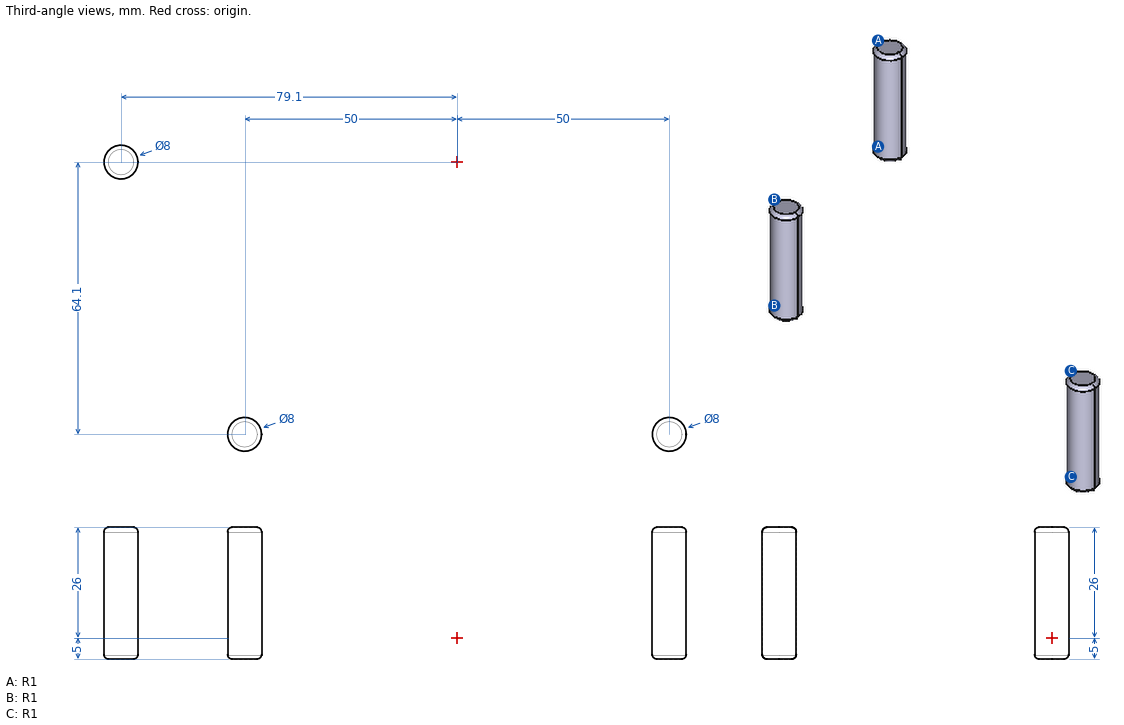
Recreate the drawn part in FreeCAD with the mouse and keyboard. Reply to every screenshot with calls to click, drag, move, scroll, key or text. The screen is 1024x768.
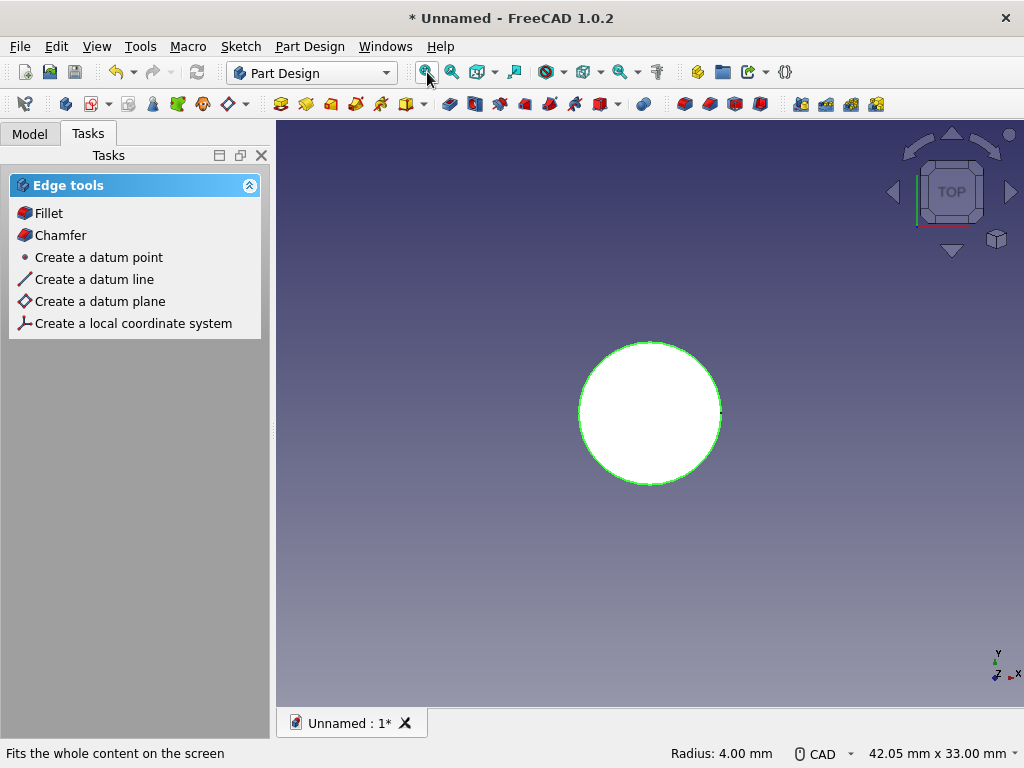
key(1)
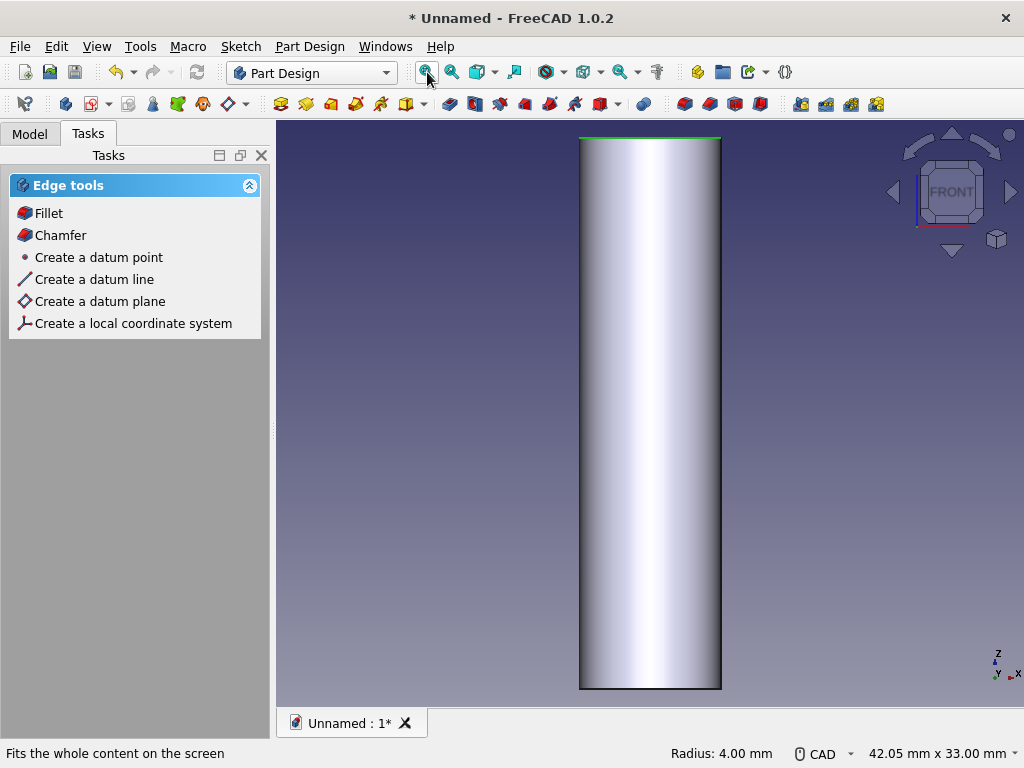
key(3)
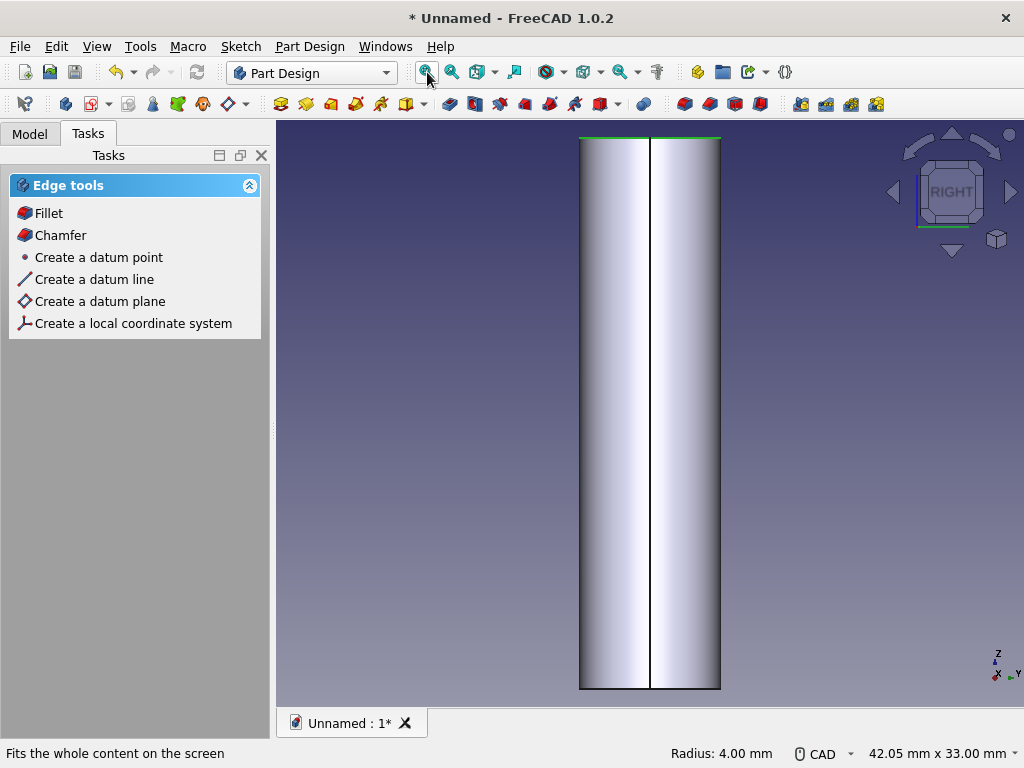
key(5)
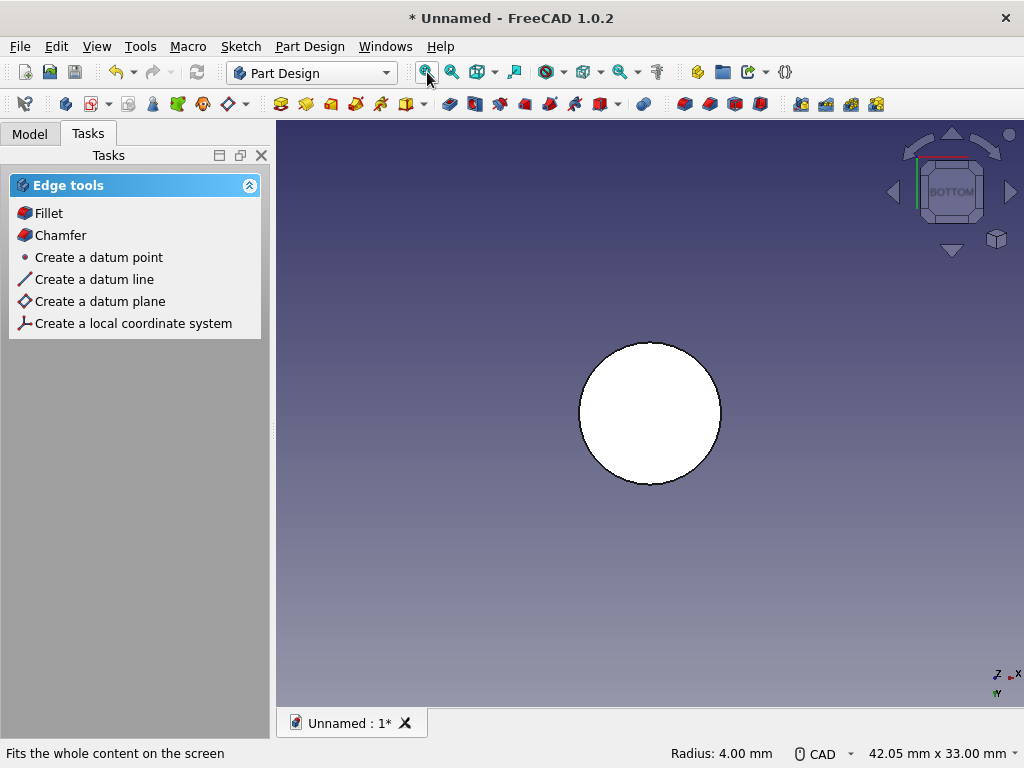
click(427, 72)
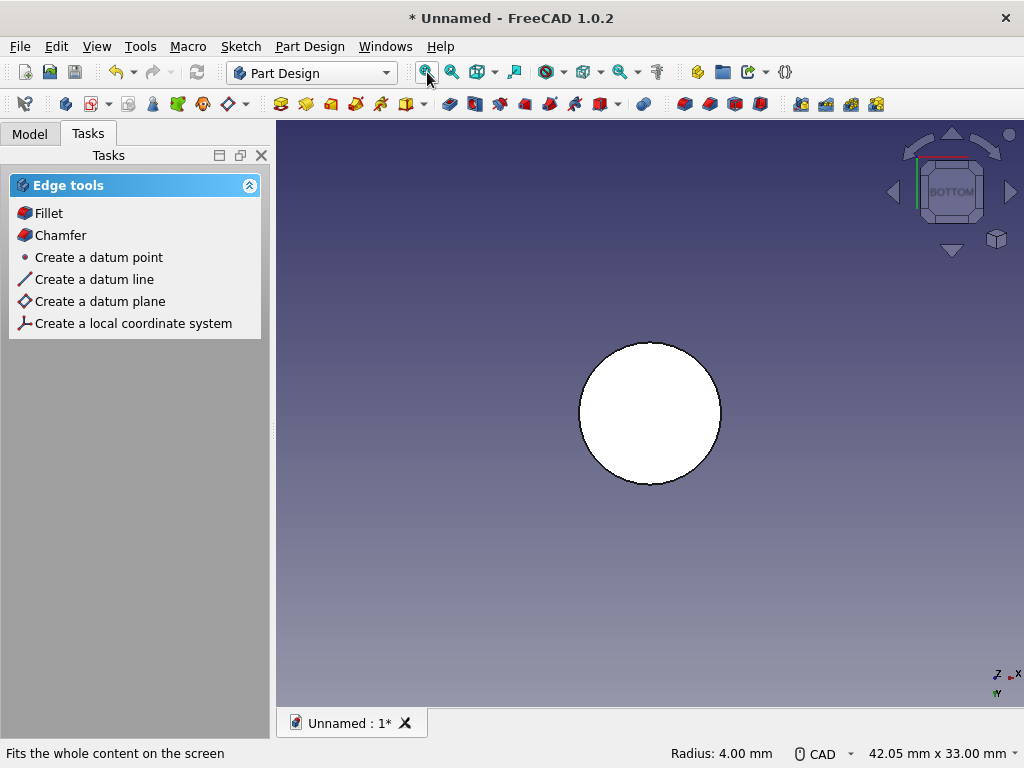
click(579, 412, ctrl)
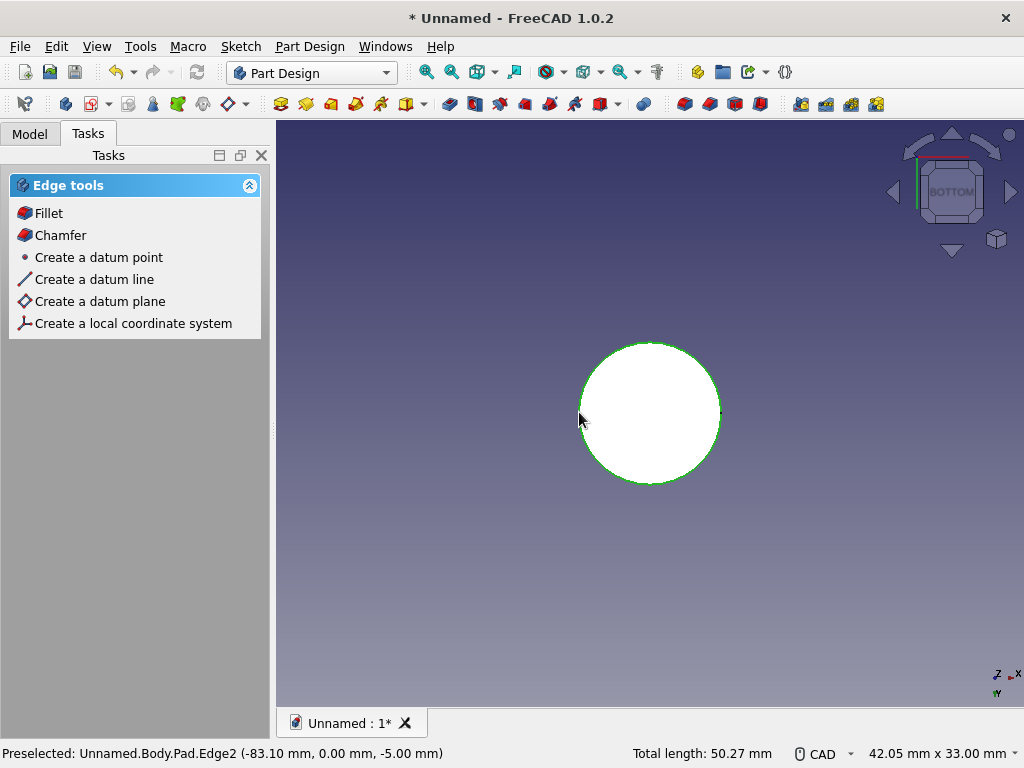
click(685, 104)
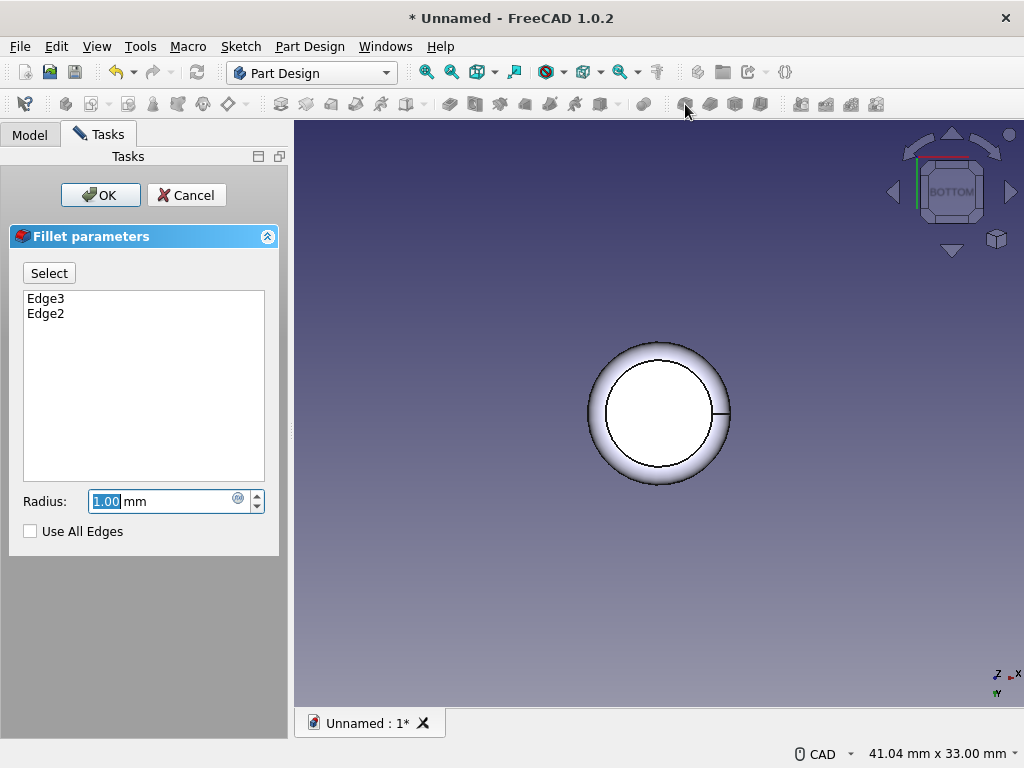
text(1)
key(Tab)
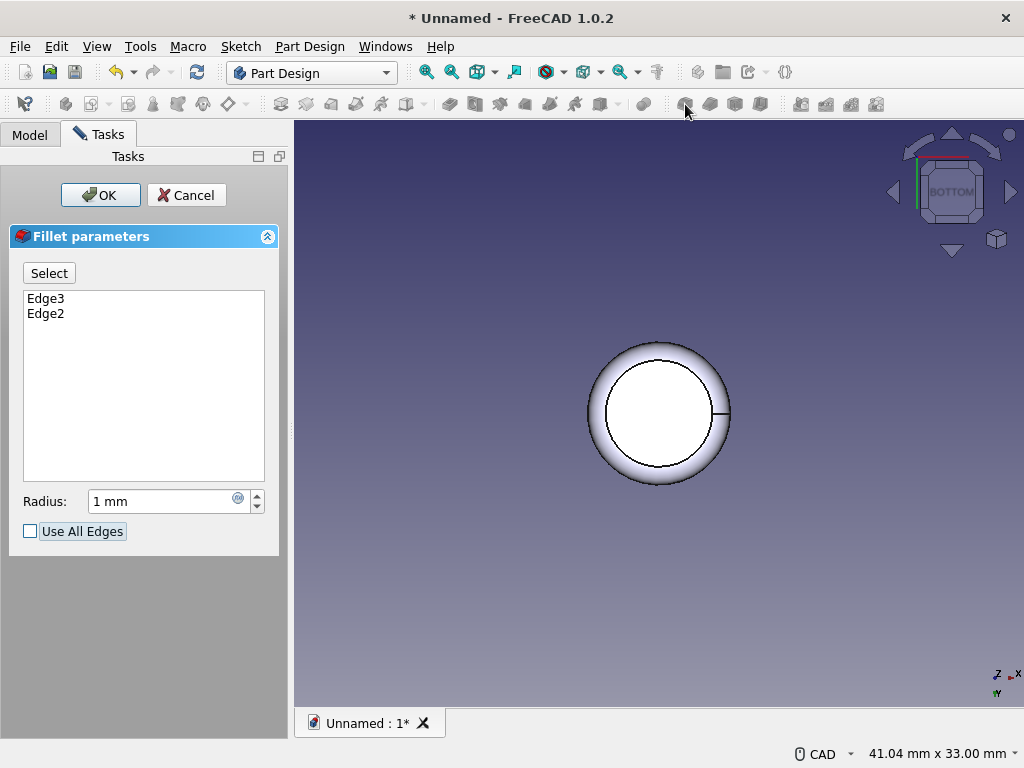
click(101, 195)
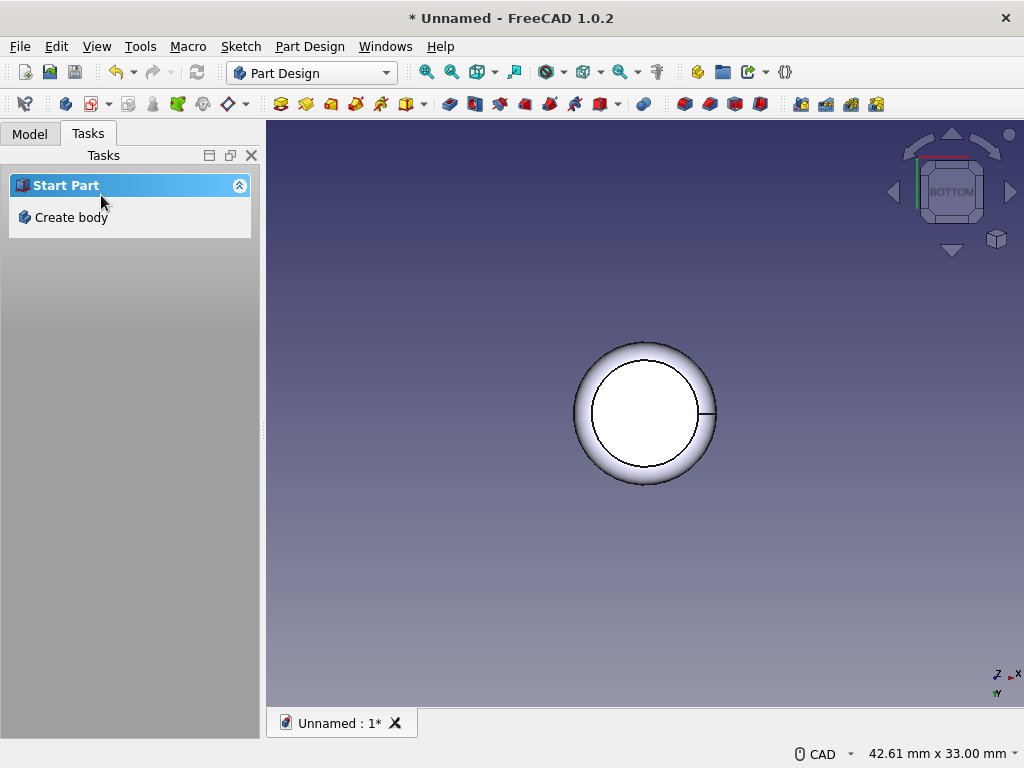
click(427, 72)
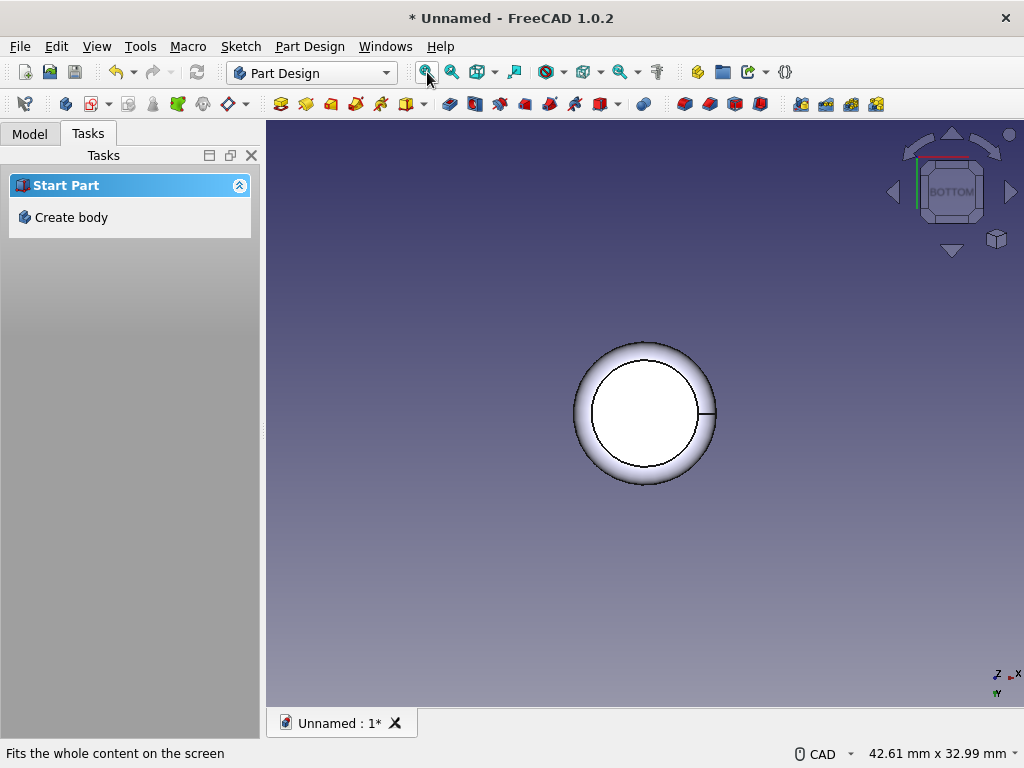
click(66, 104)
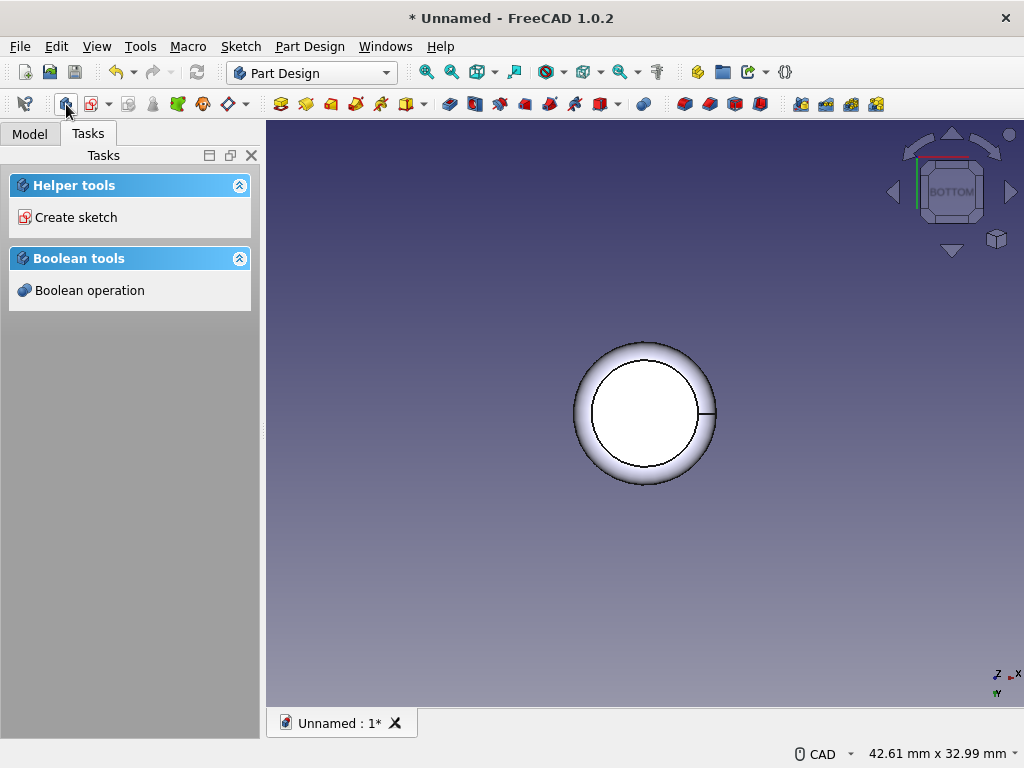
click(306, 667)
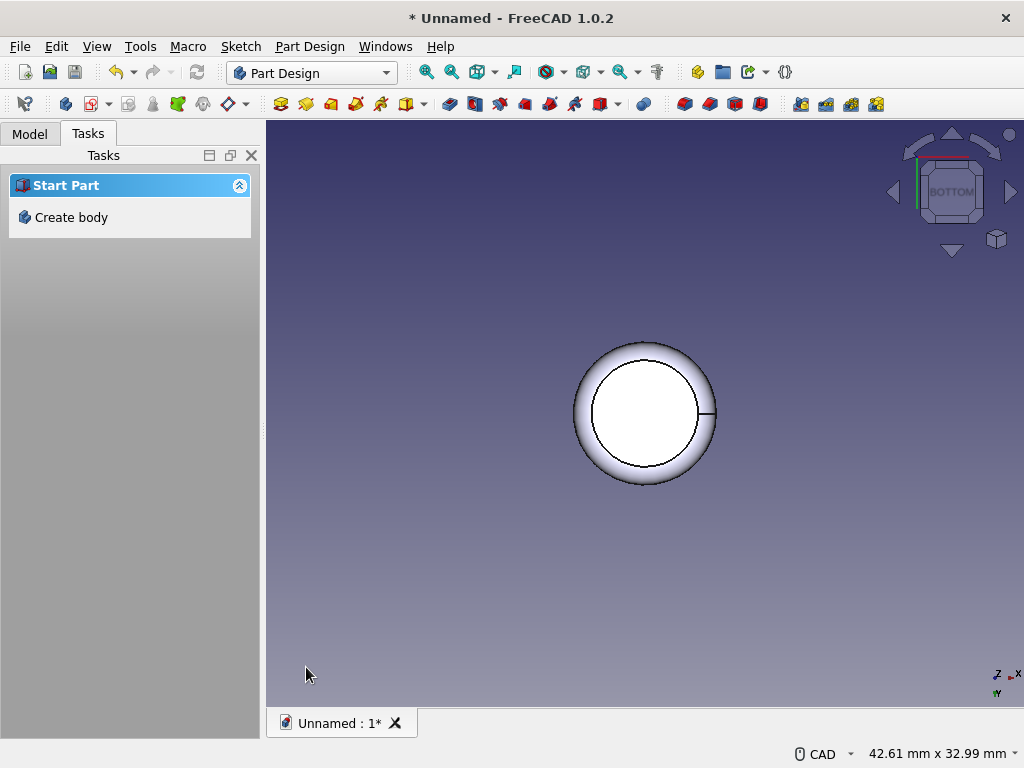
click(90, 104)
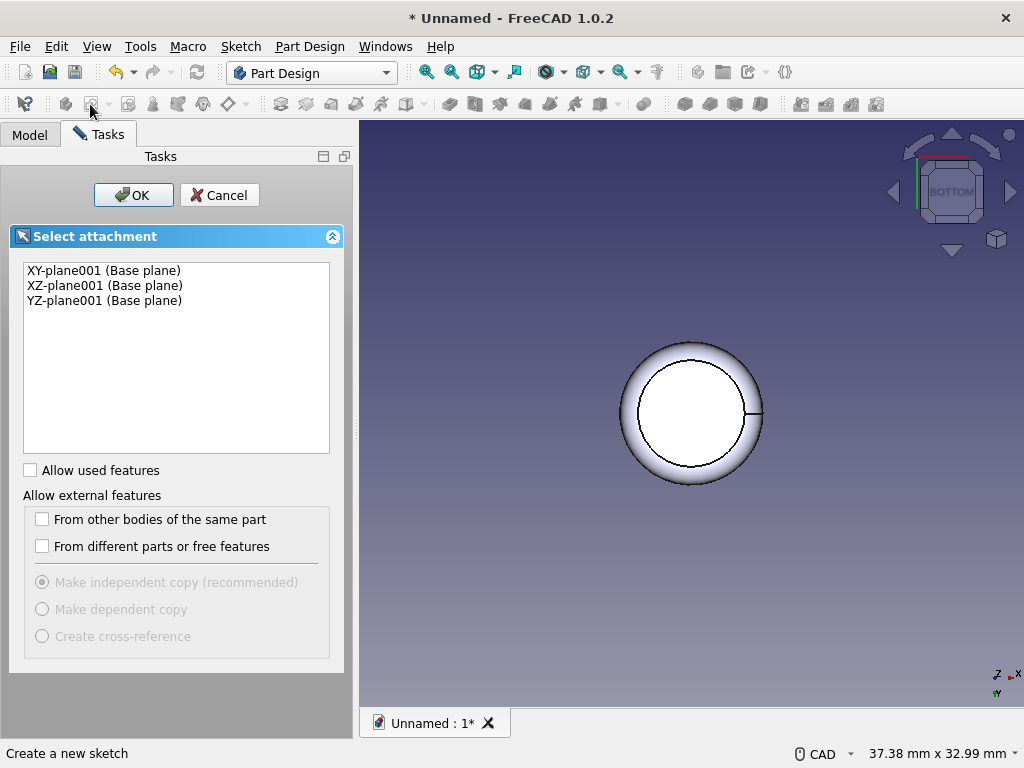
click(84, 270)